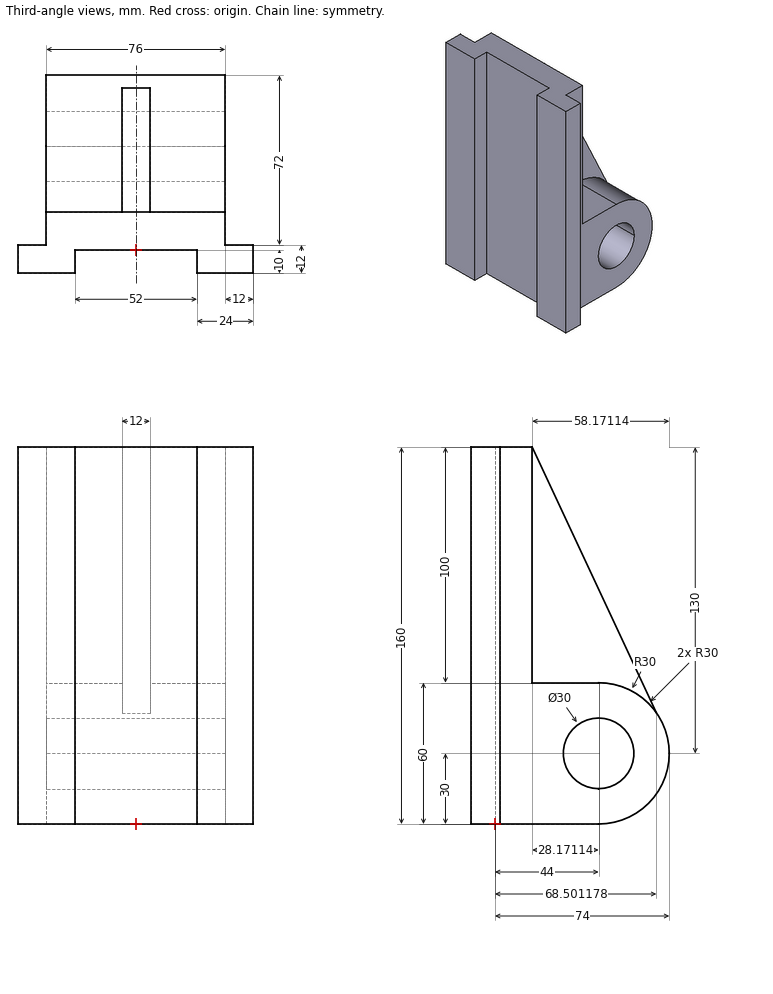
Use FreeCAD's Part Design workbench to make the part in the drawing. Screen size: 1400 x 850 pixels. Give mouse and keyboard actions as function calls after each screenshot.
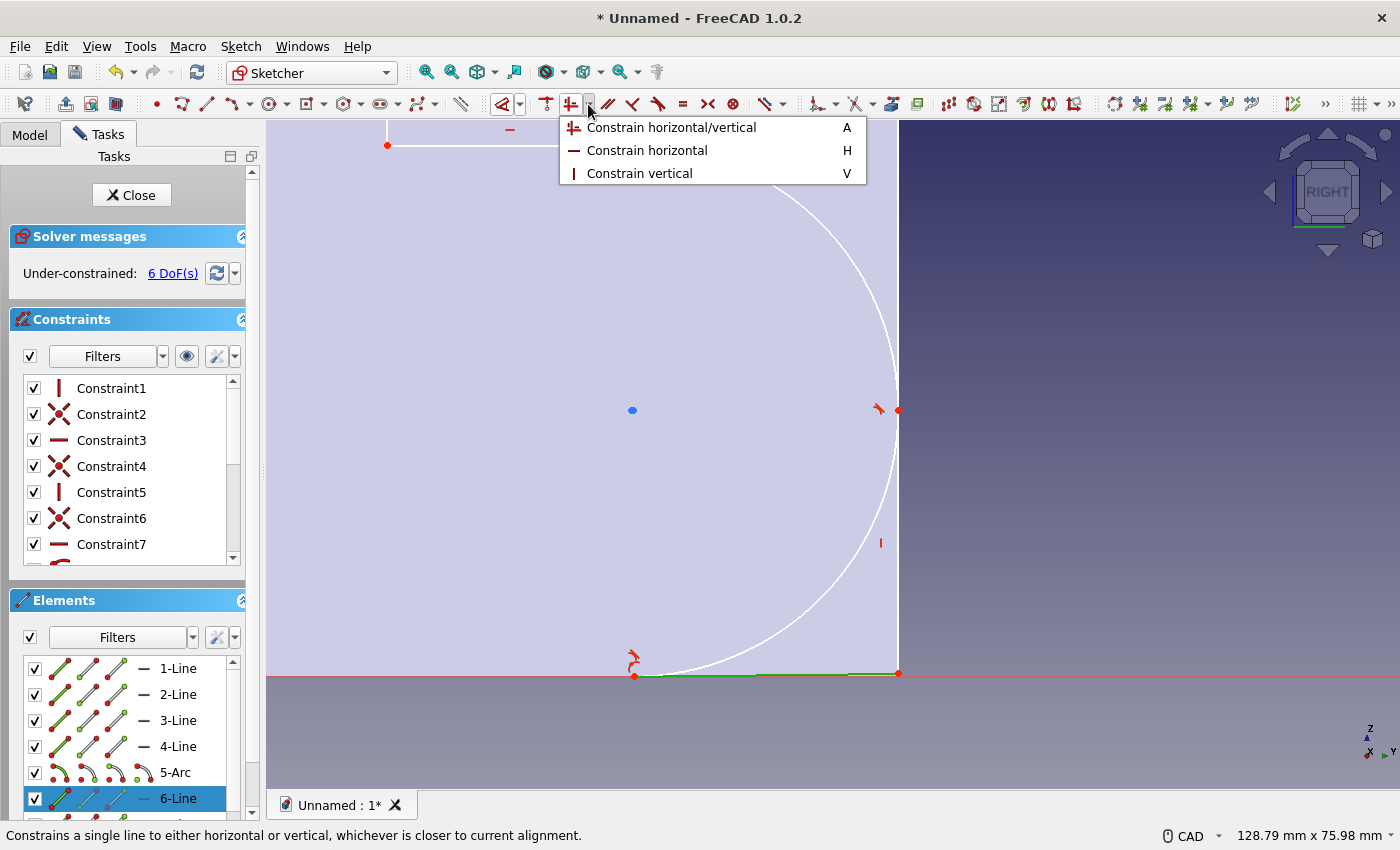
click(713, 150)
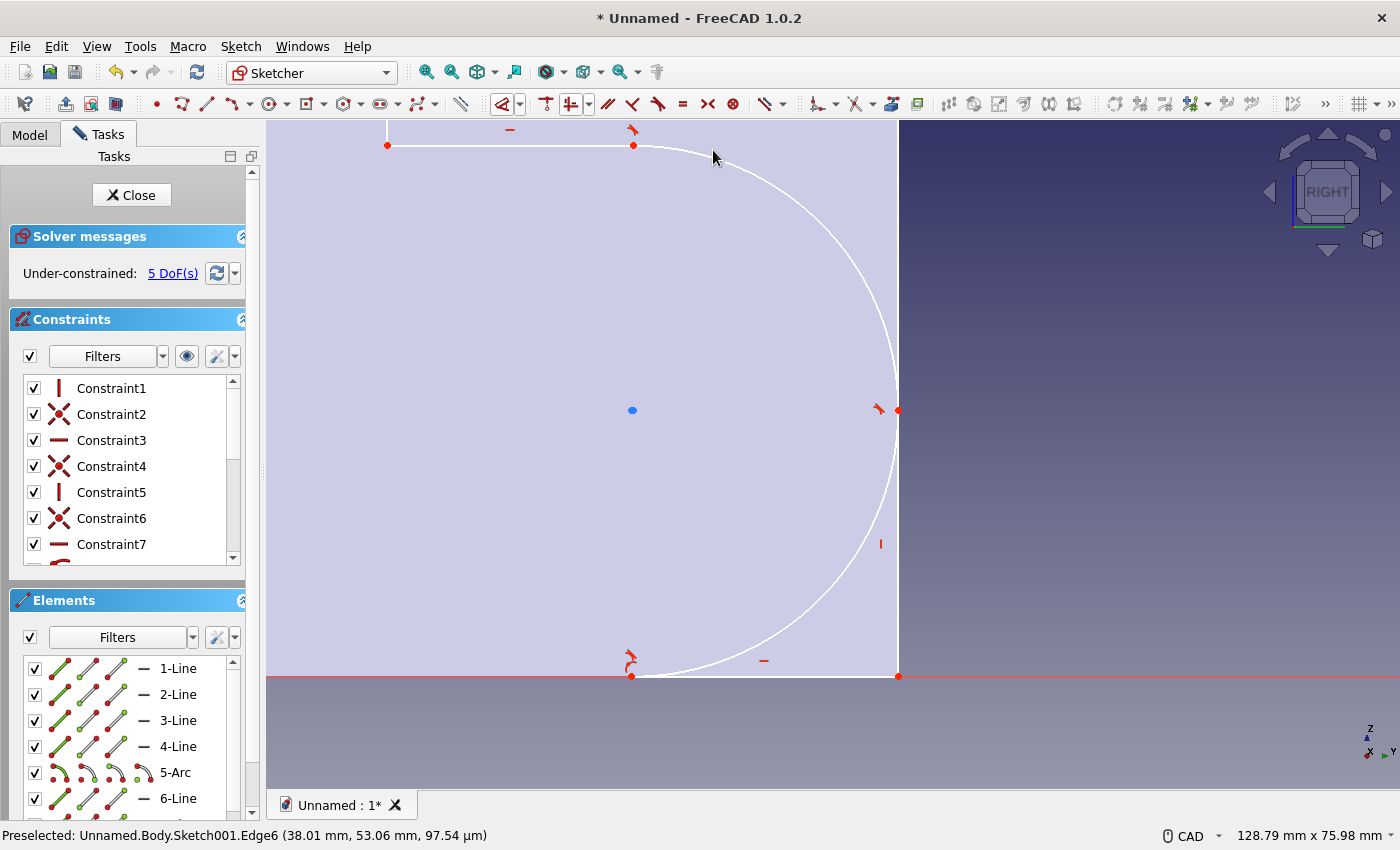
click(869, 290)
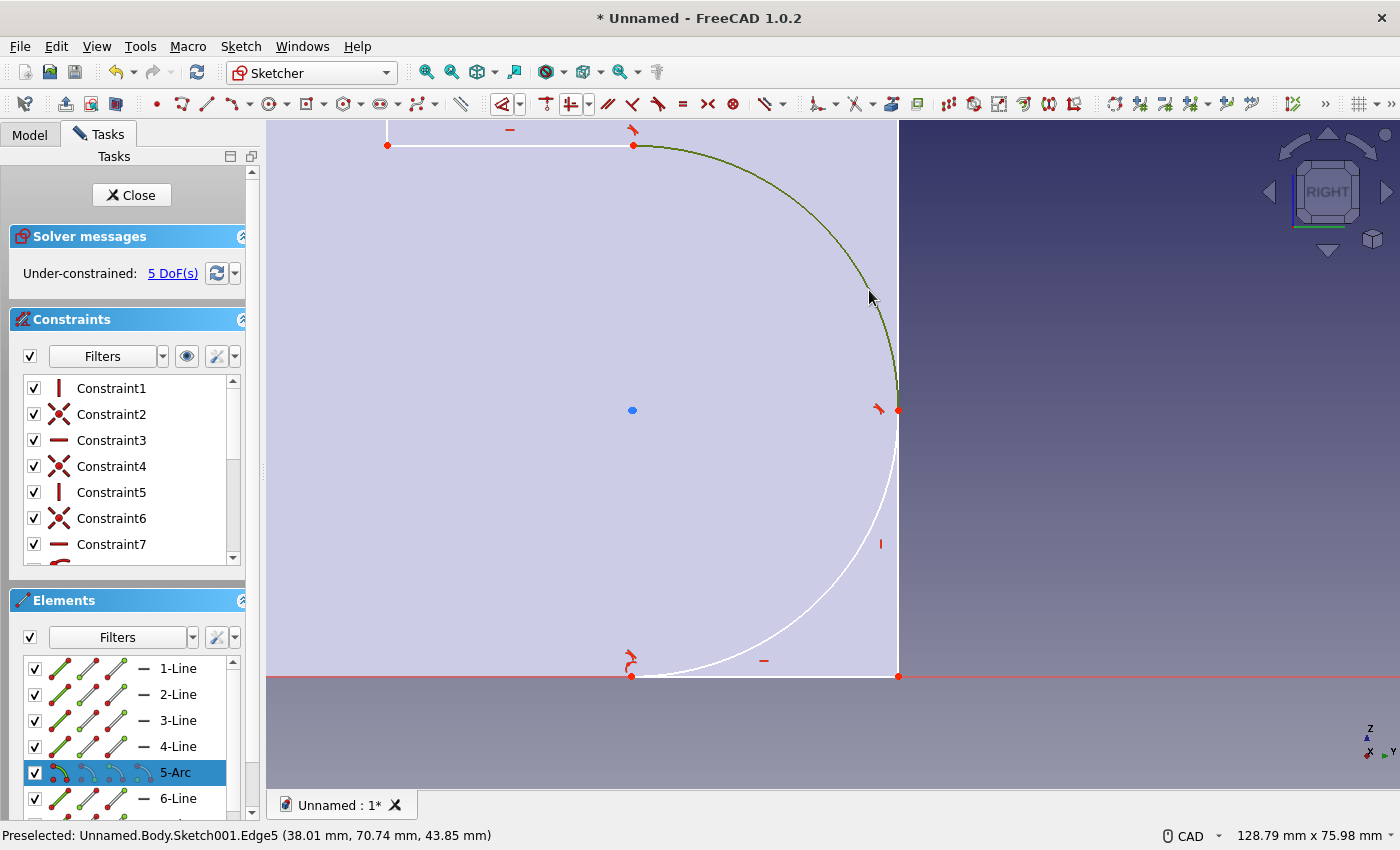
click(753, 648)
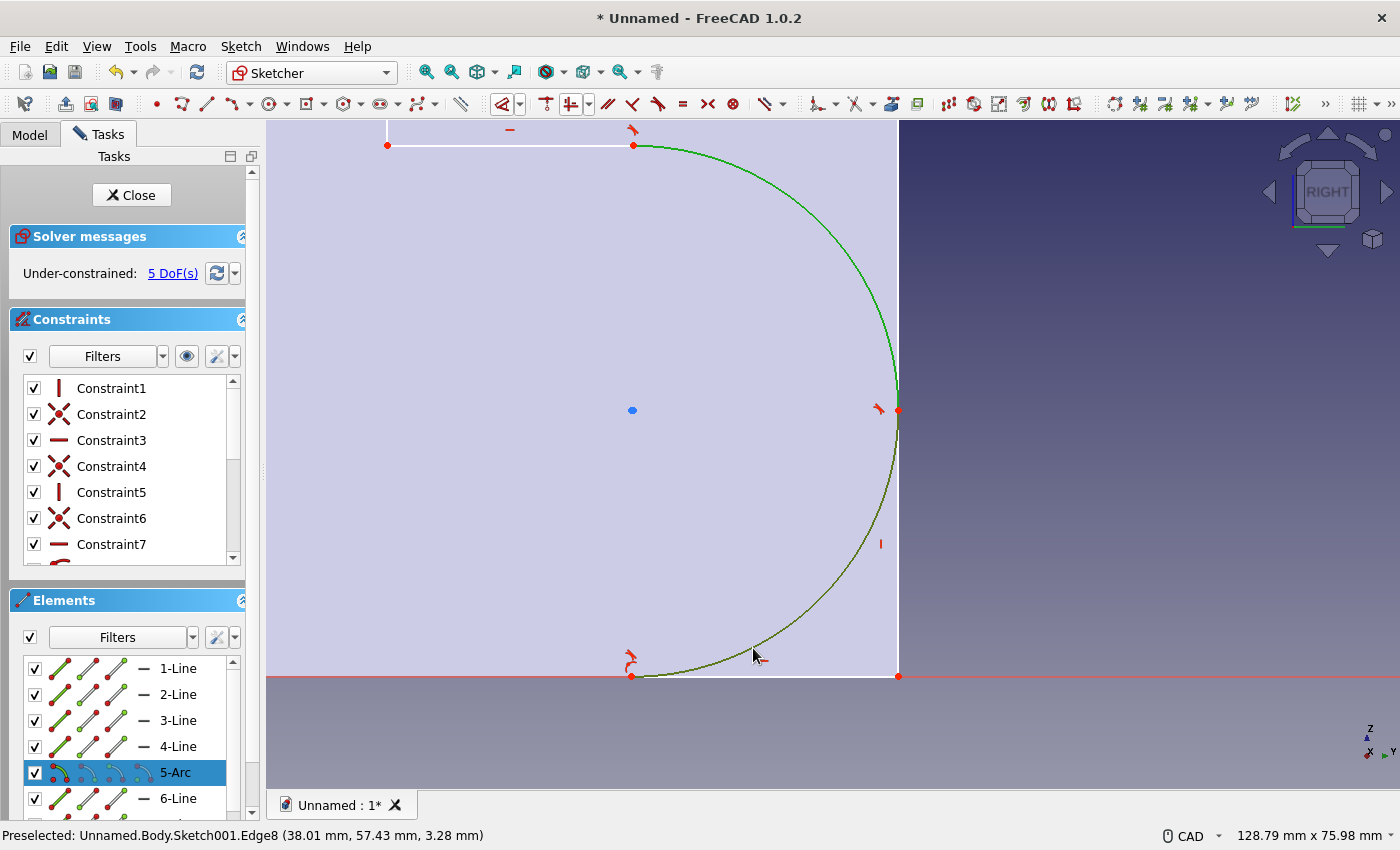
click(683, 104)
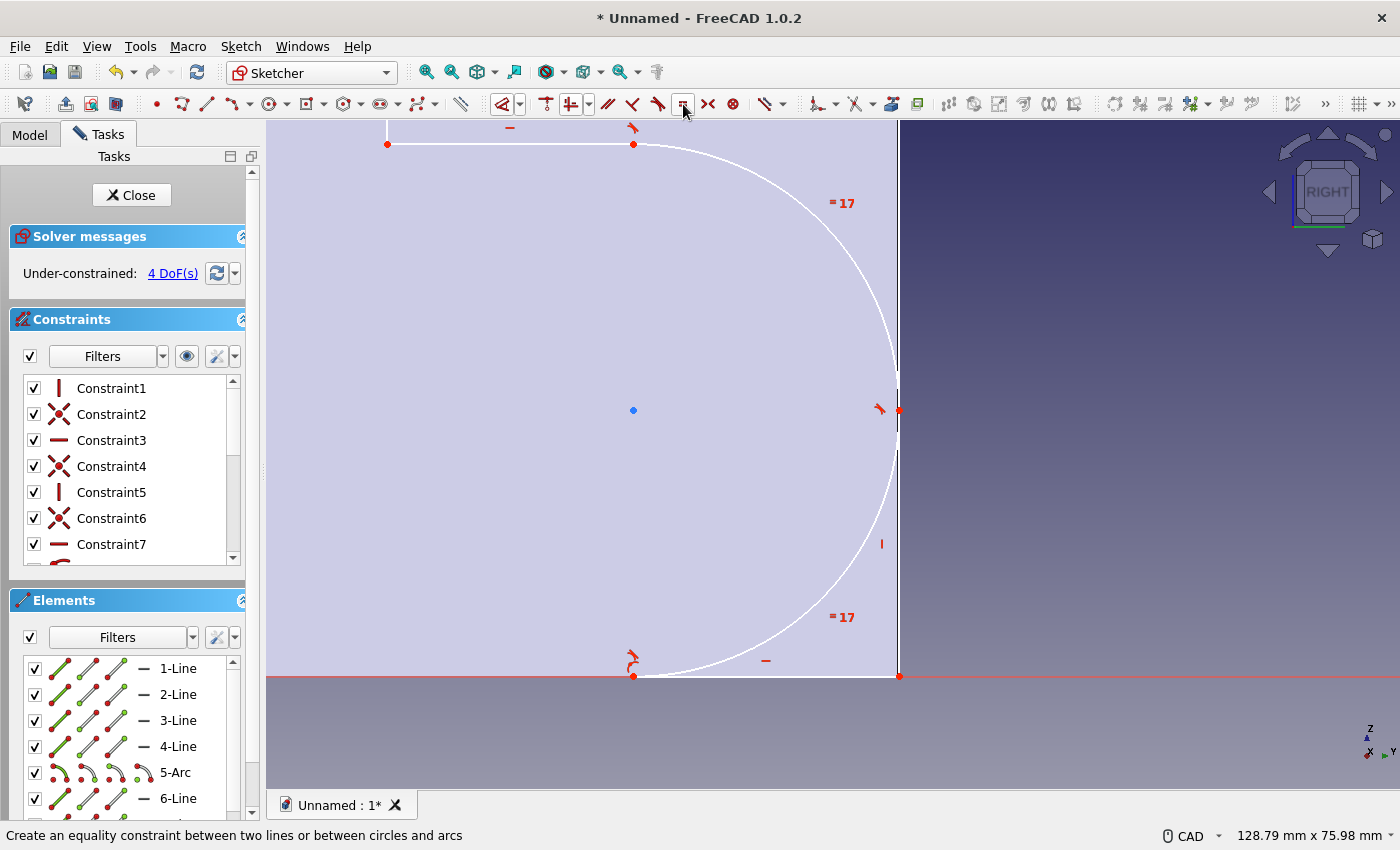
click(502, 104)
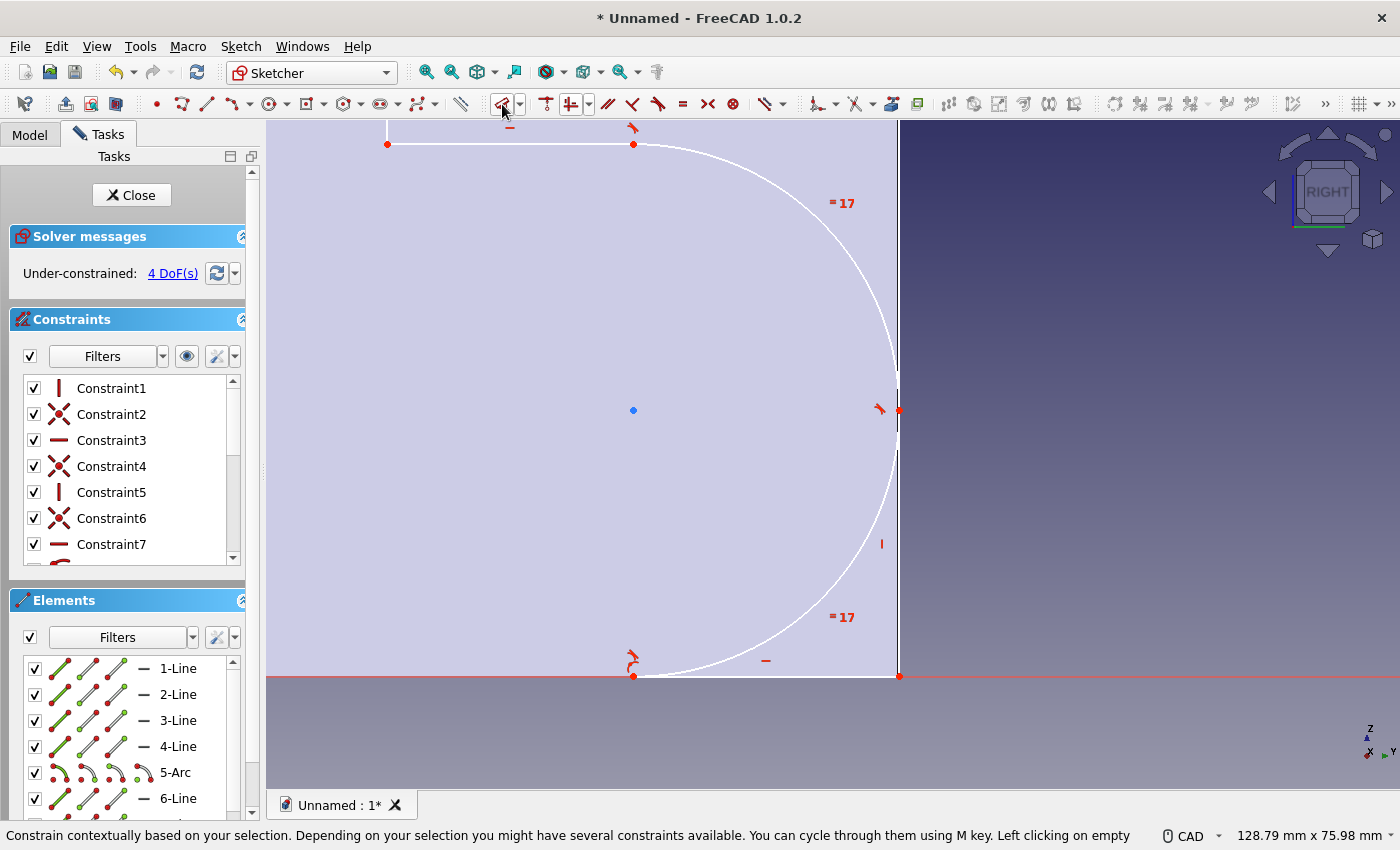
click(870, 290)
click(931, 419)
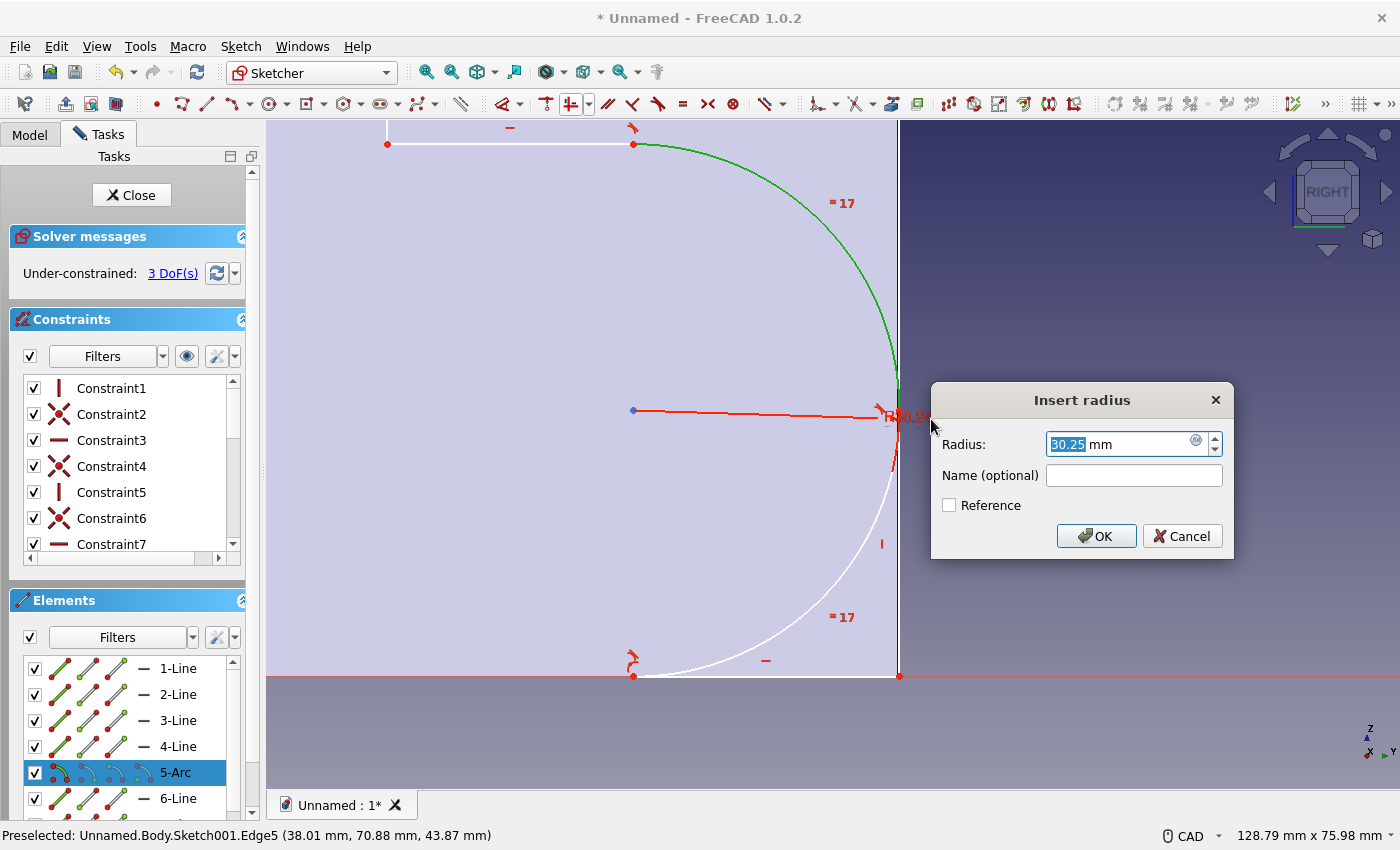
text(30)
key(Return)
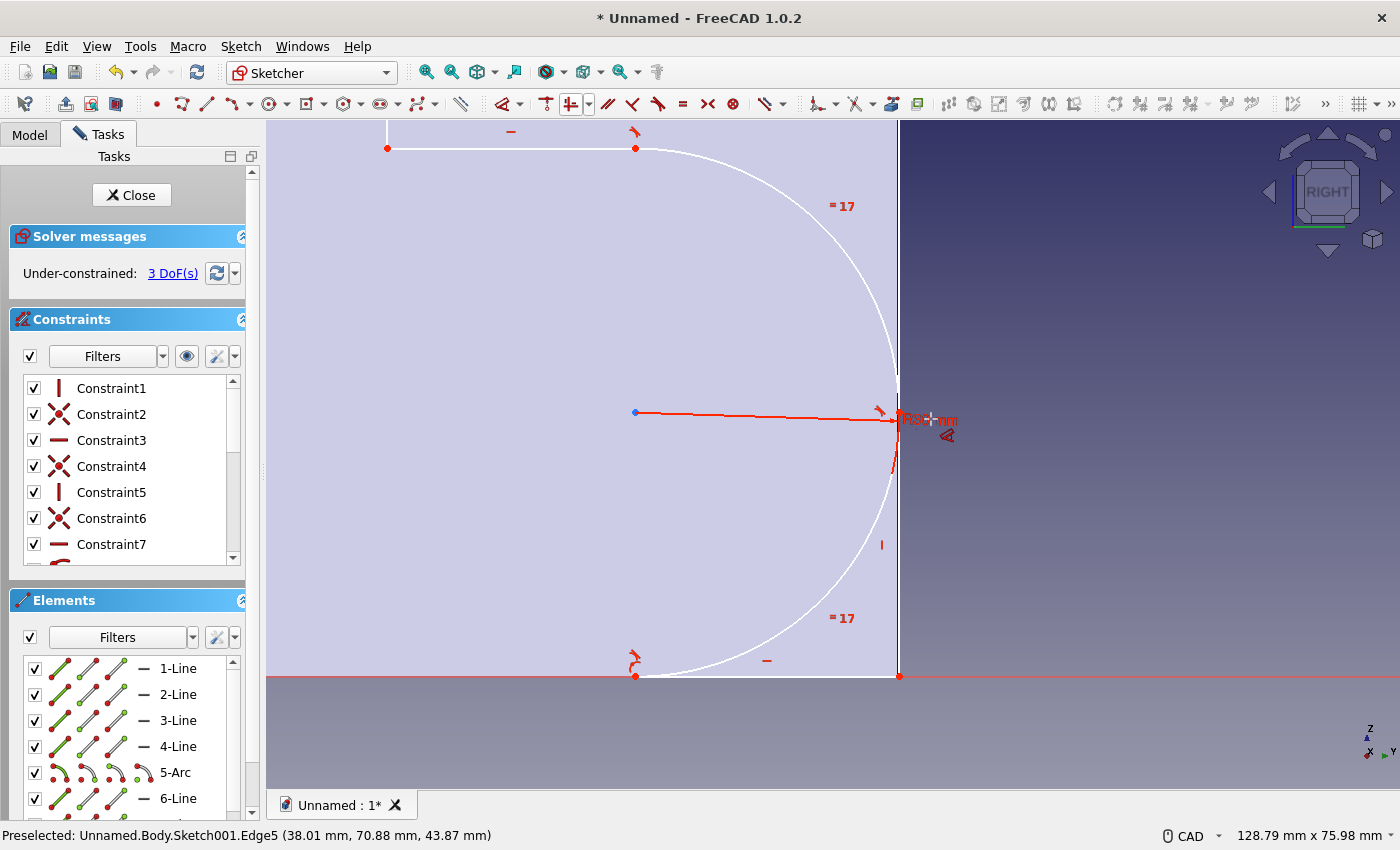
click(899, 184)
click(933, 280)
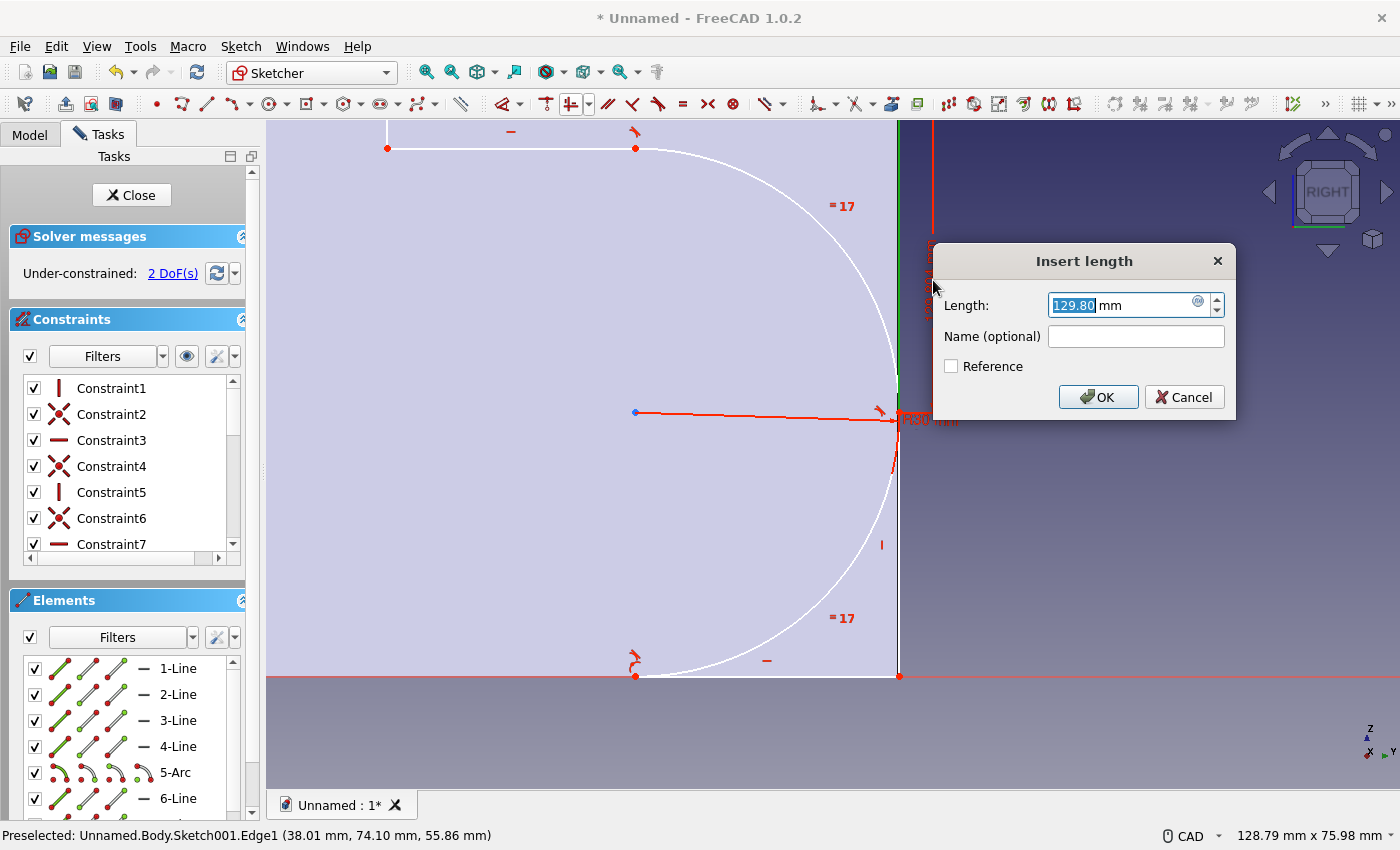
text(130)
key(Return)